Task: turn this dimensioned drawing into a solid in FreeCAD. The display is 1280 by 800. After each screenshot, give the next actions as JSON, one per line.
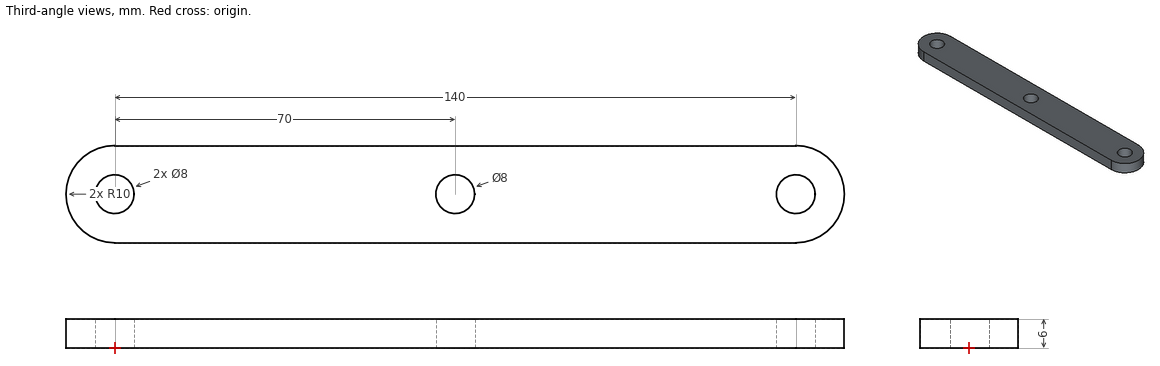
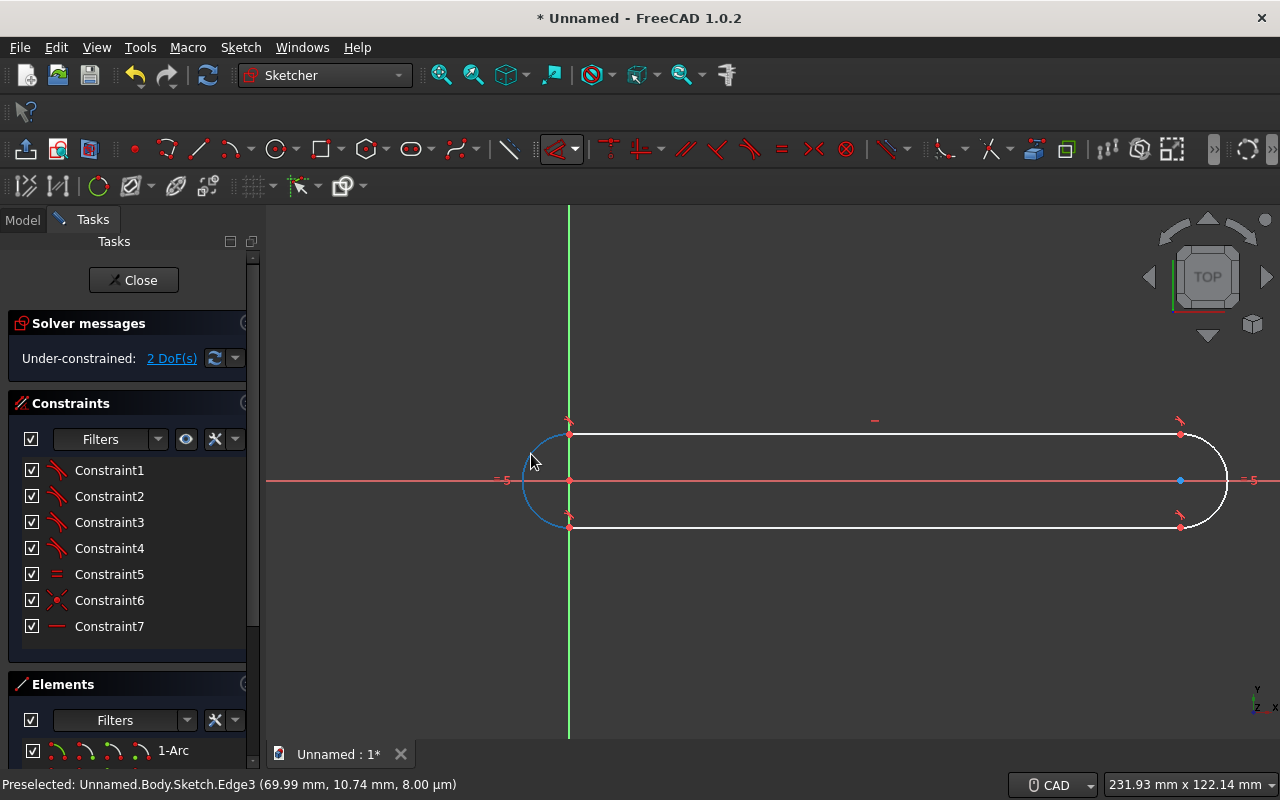
{"action": "left_click", "coordinate": [532, 453]}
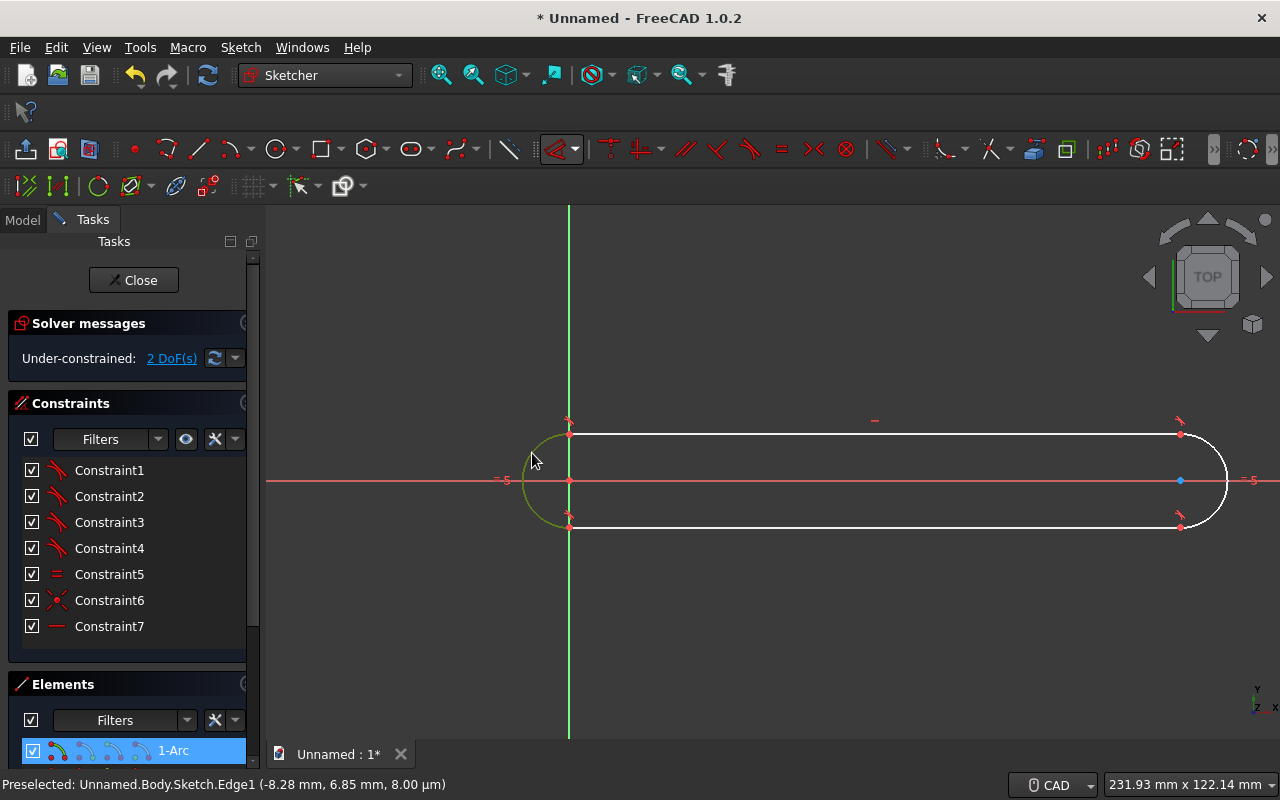
{"action": "left_click", "coordinate": [578, 150]}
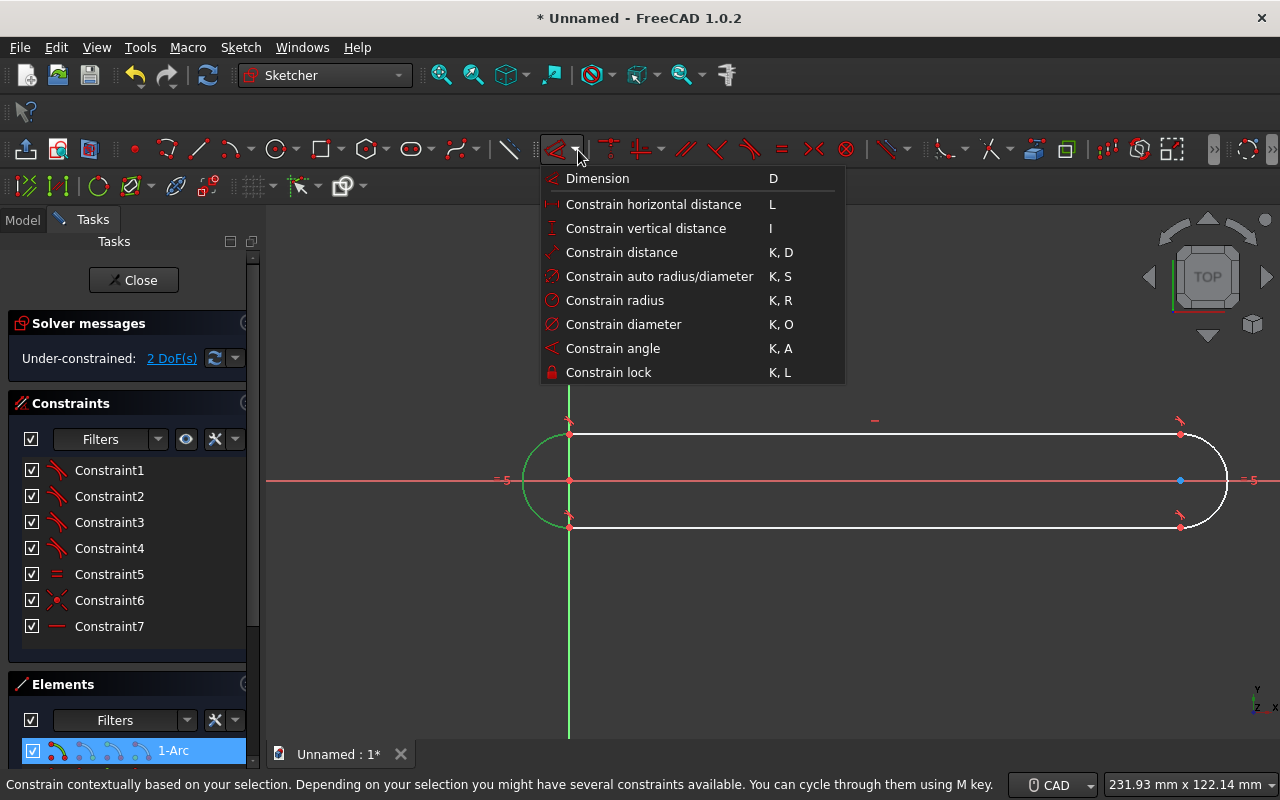
{"action": "left_click", "coordinate": [693, 300]}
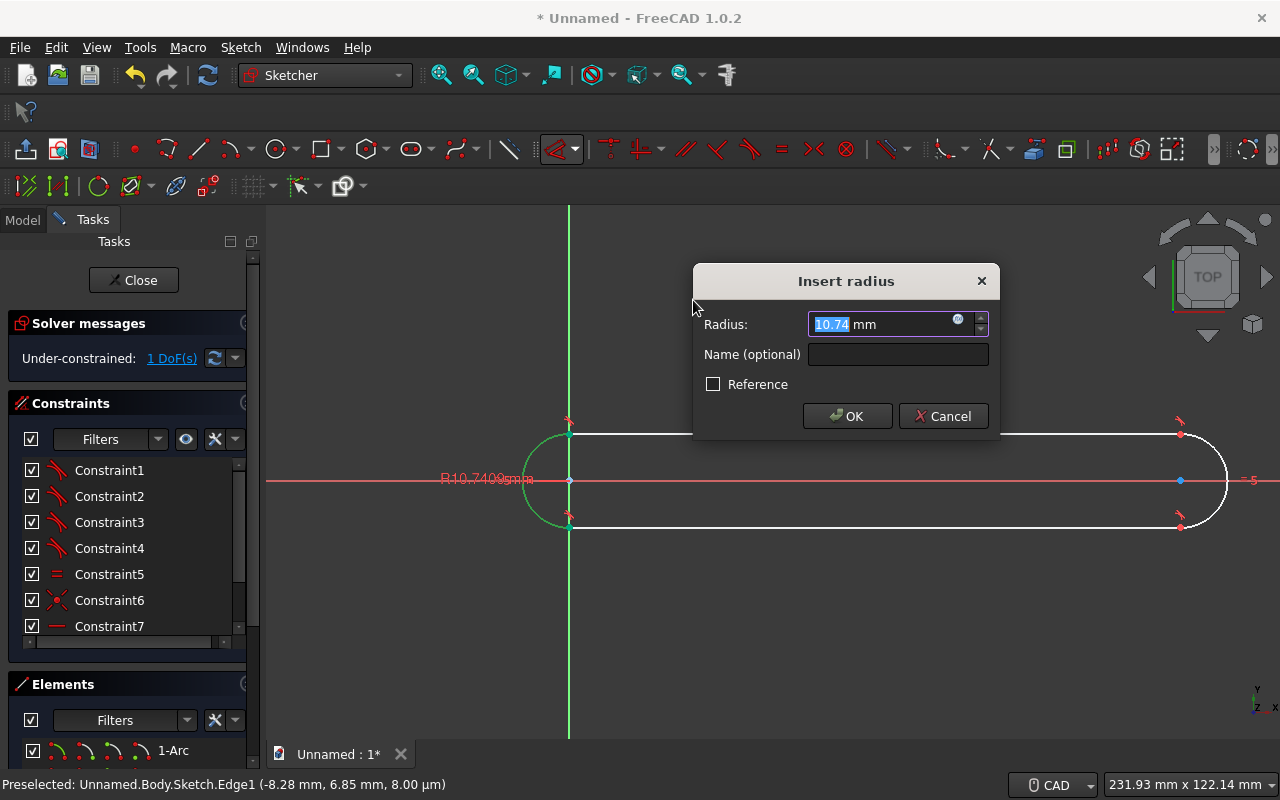
{"action": "type", "text": "10"}
{"action": "key", "text": "Return"}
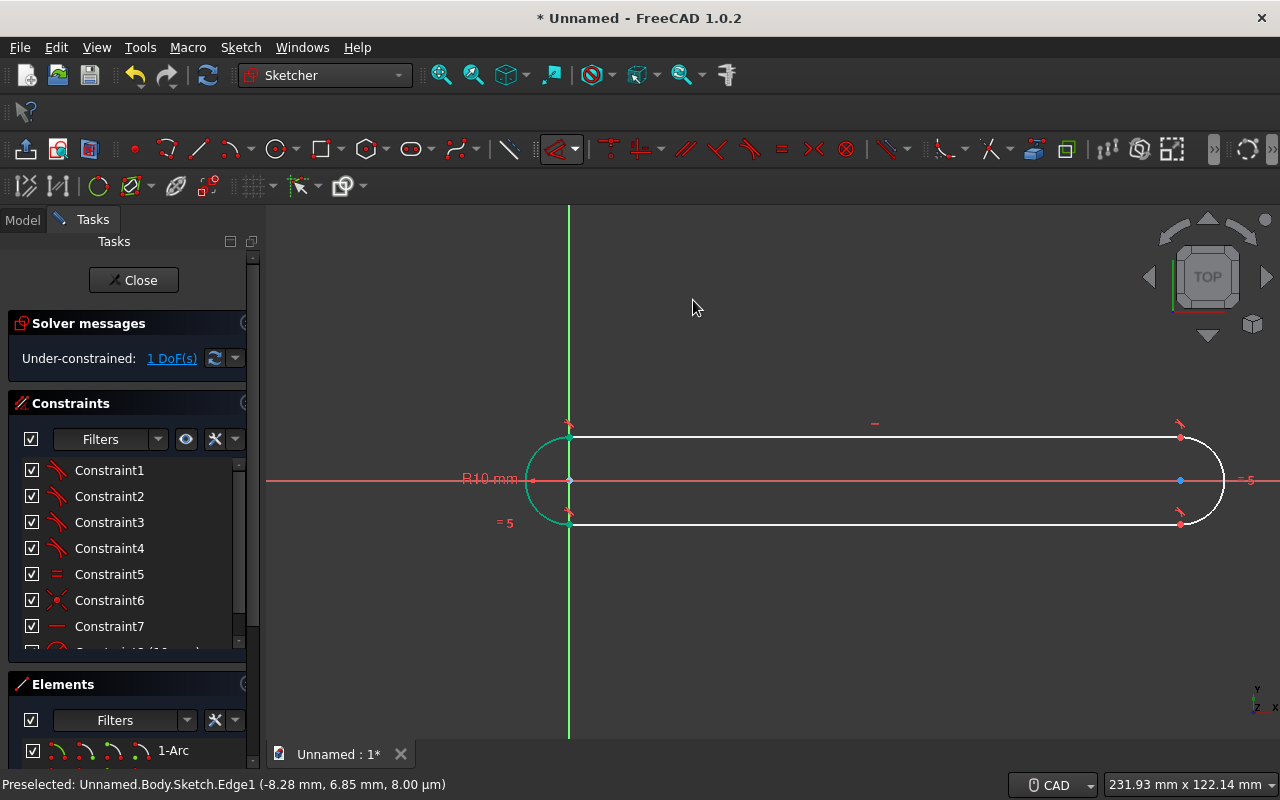
{"action": "left_click", "coordinate": [753, 437]}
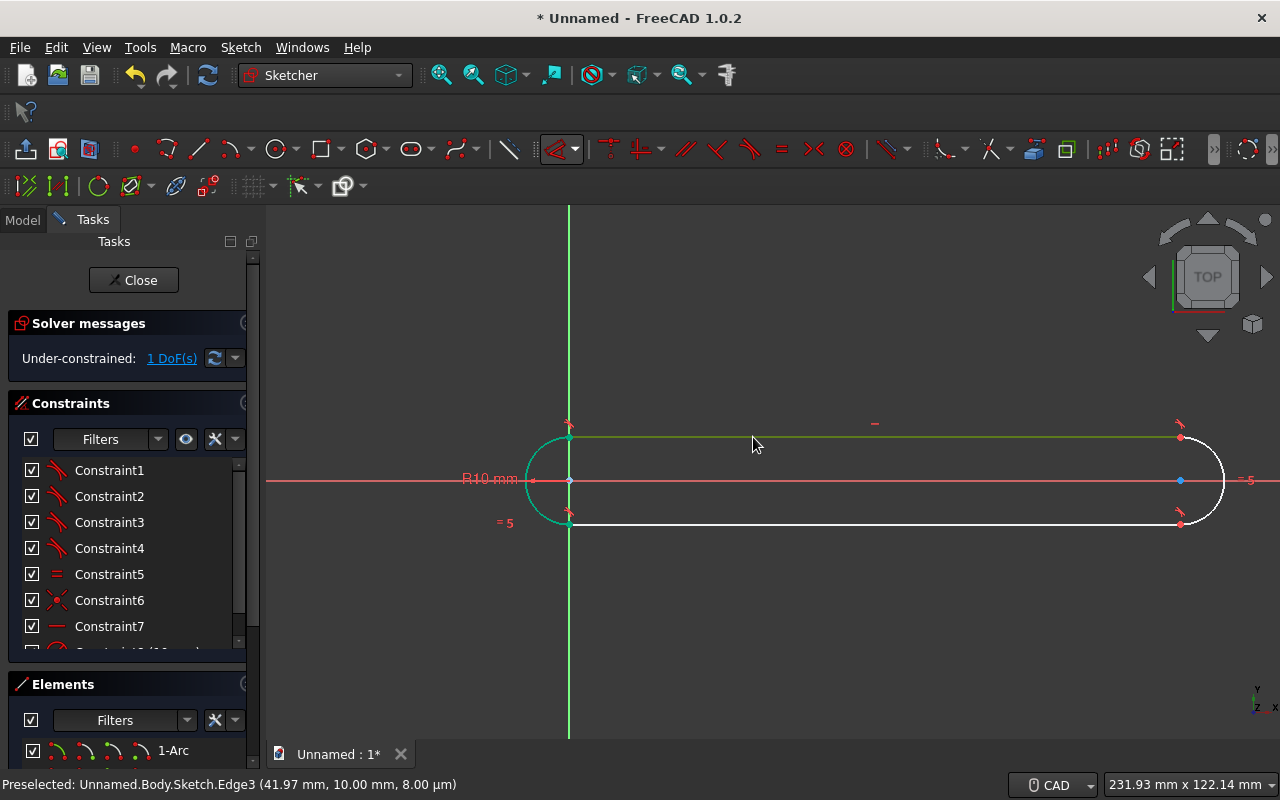
{"action": "left_click", "coordinate": [578, 150]}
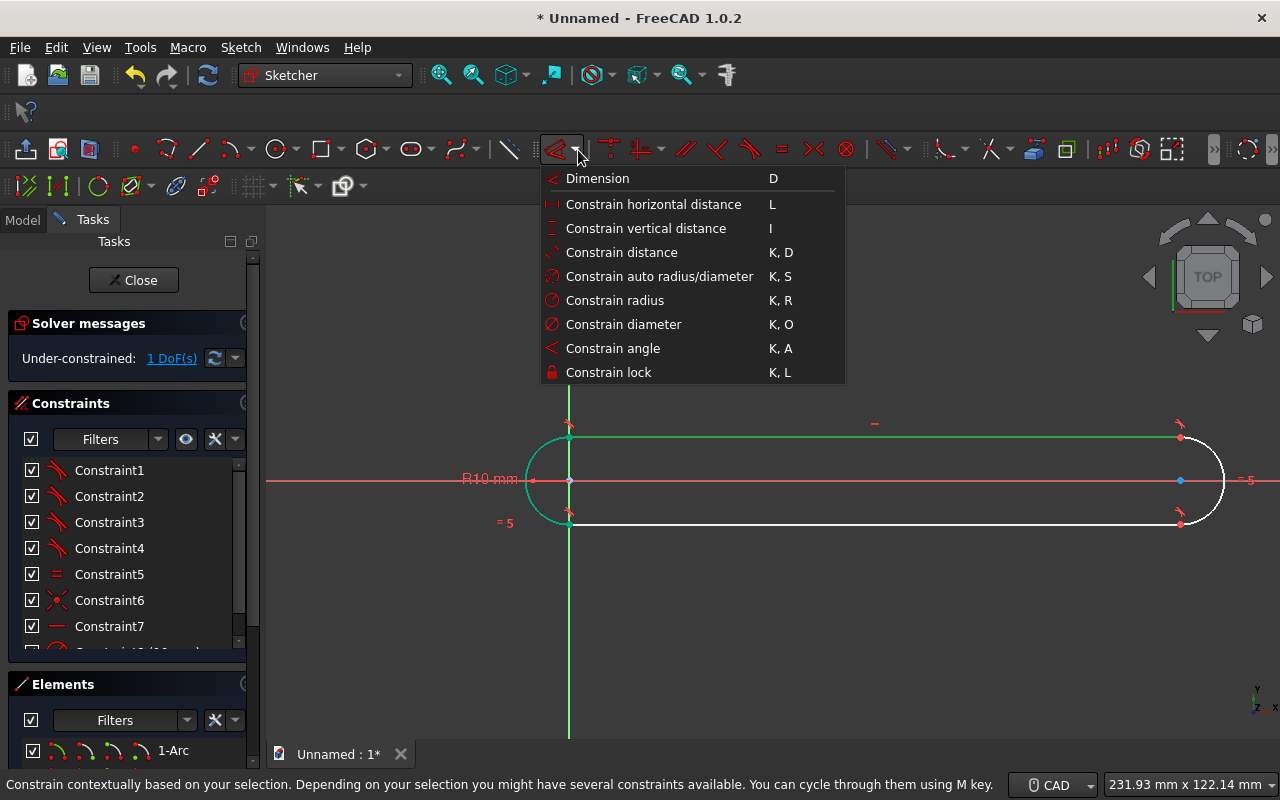
{"action": "left_click", "coordinate": [693, 204]}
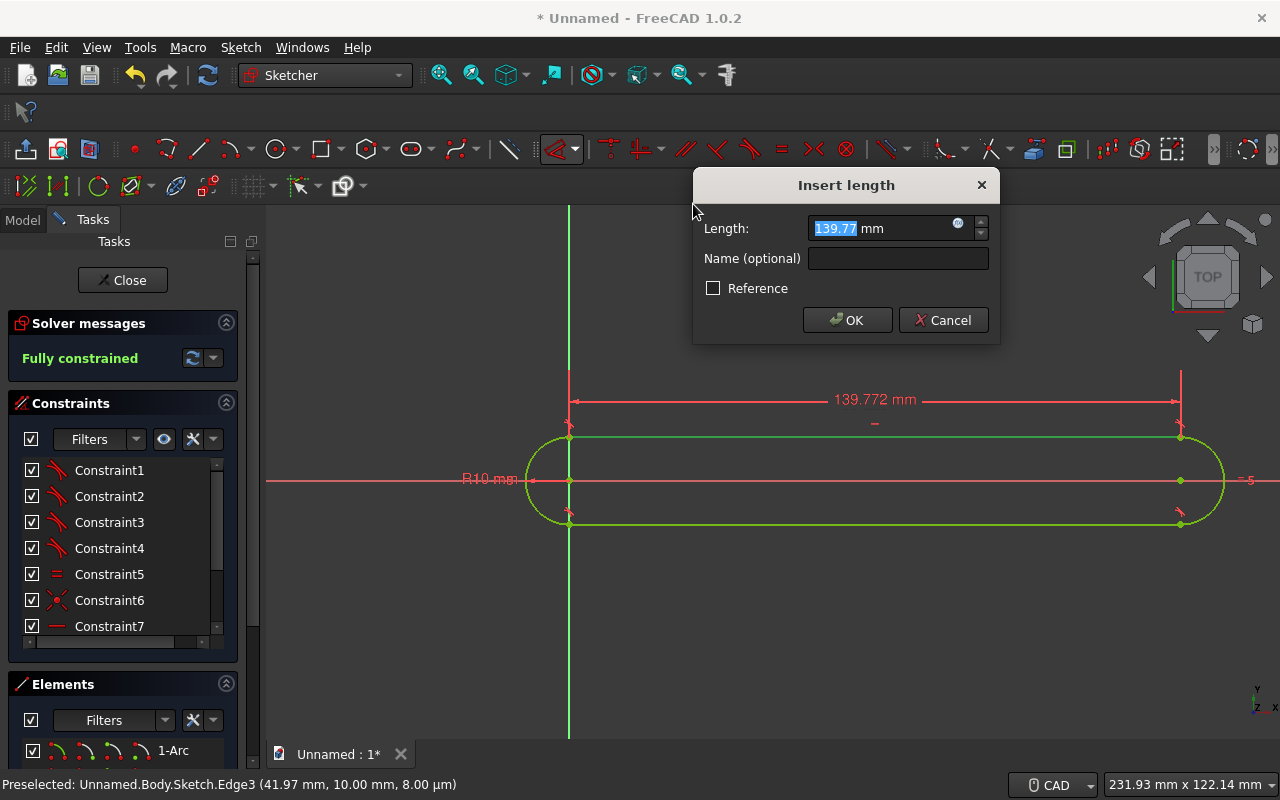
{"action": "type", "text": "140"}
{"action": "key", "text": "Return"}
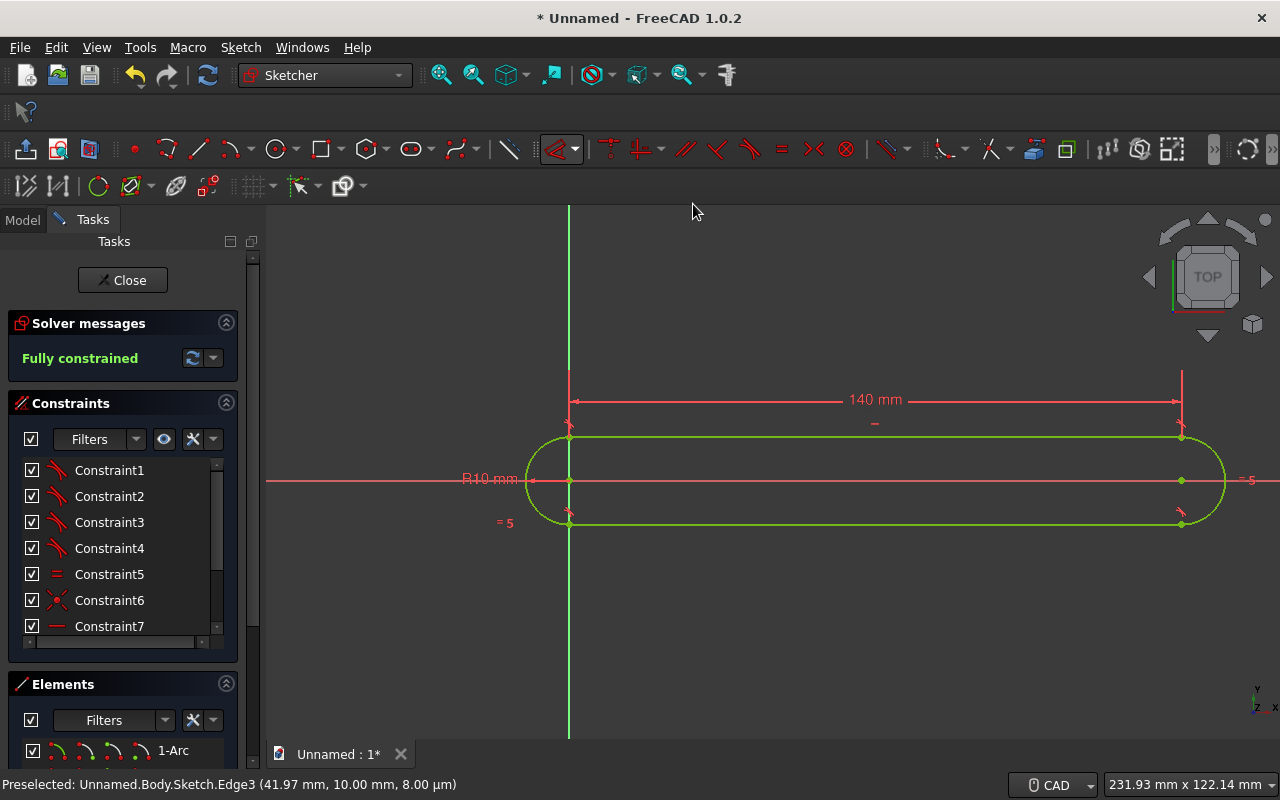
{"action": "left_click", "coordinate": [123, 280]}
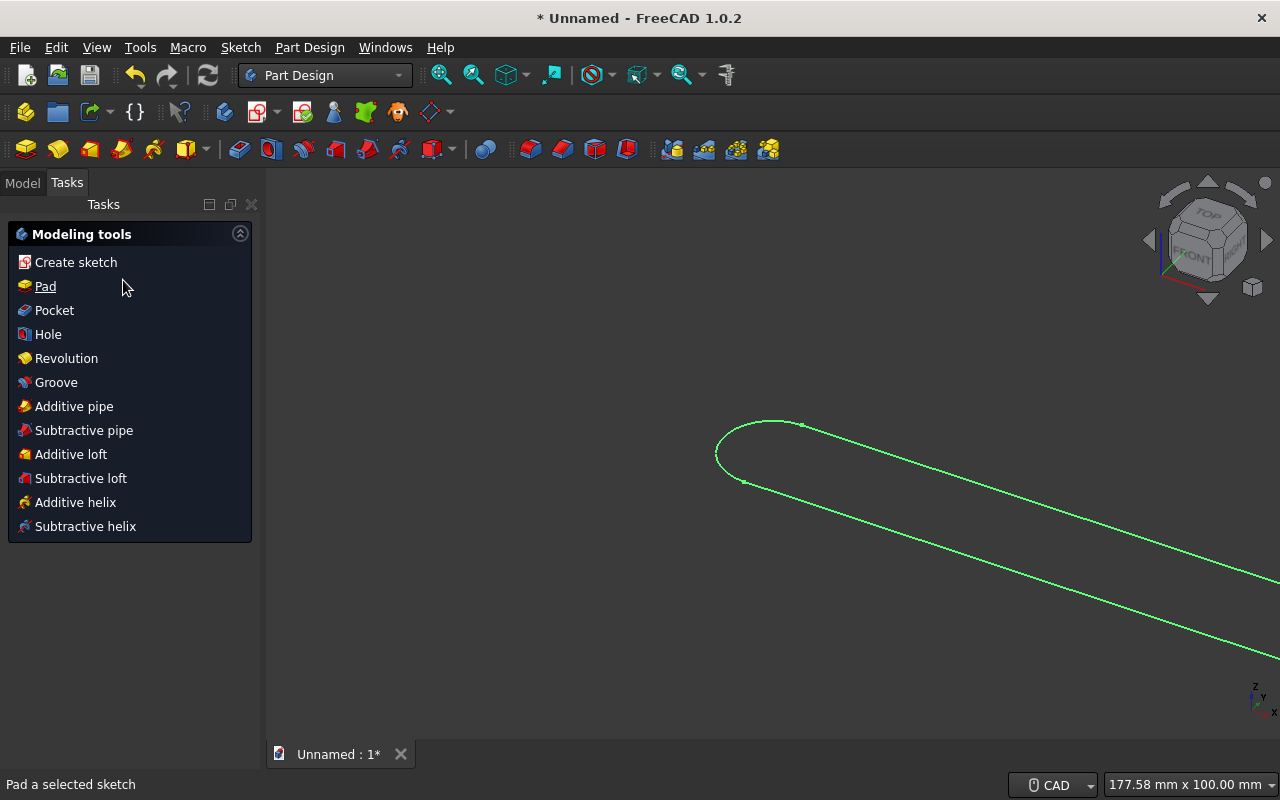
{"action": "left_click", "coordinate": [26, 150]}